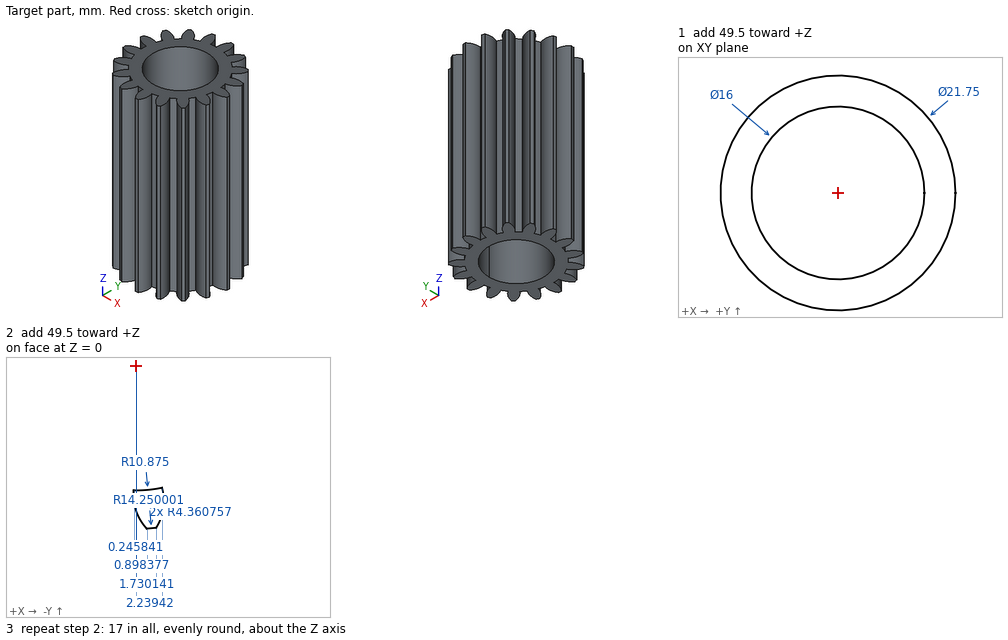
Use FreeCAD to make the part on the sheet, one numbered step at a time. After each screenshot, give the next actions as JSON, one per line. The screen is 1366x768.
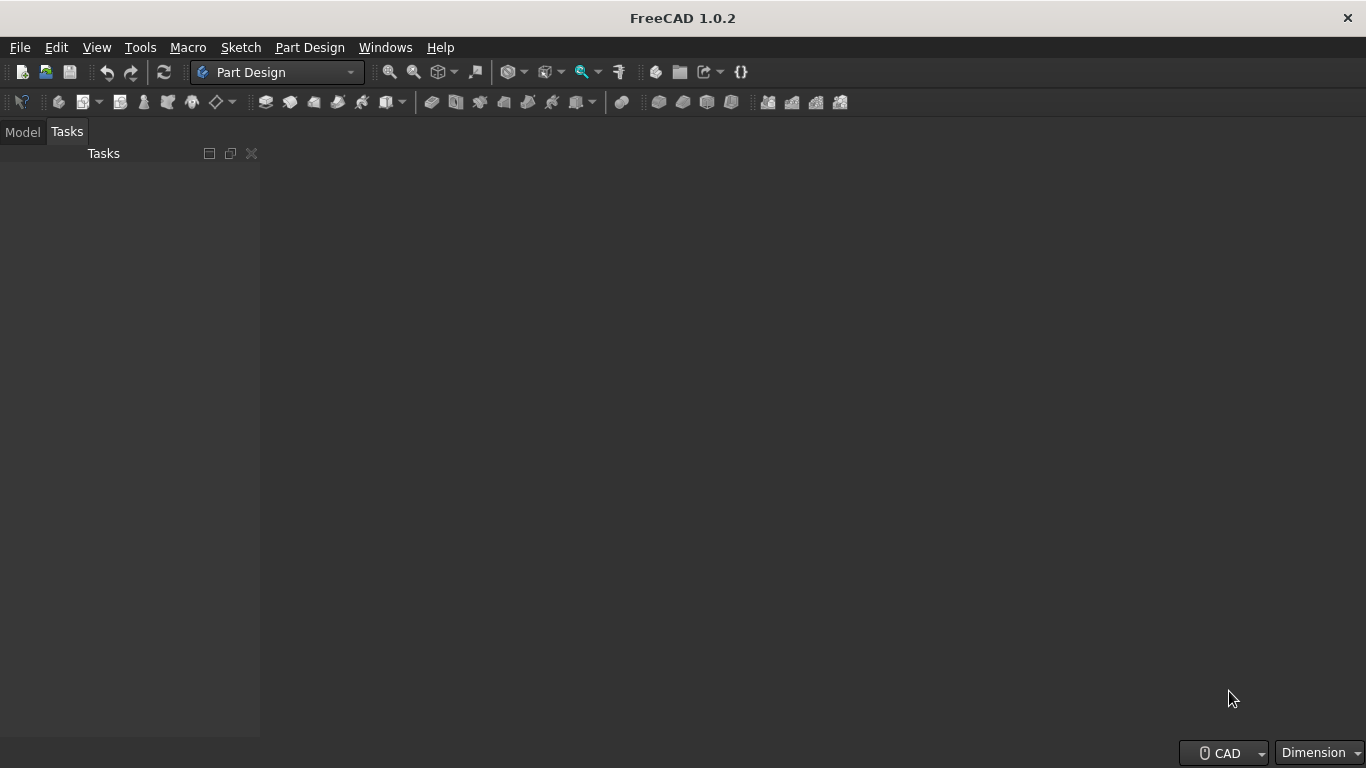
{"action": "left_click", "coordinate": [22, 72]}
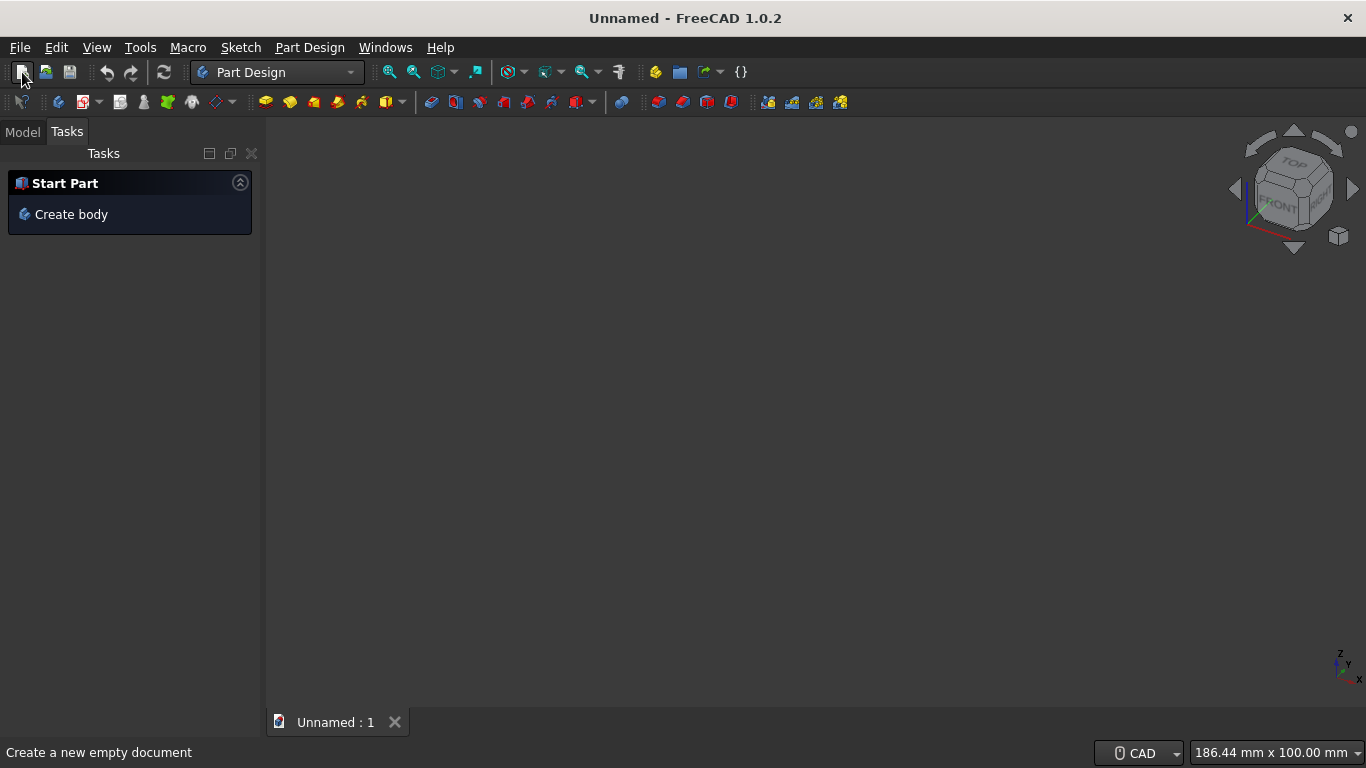
{"action": "left_click", "coordinate": [84, 102]}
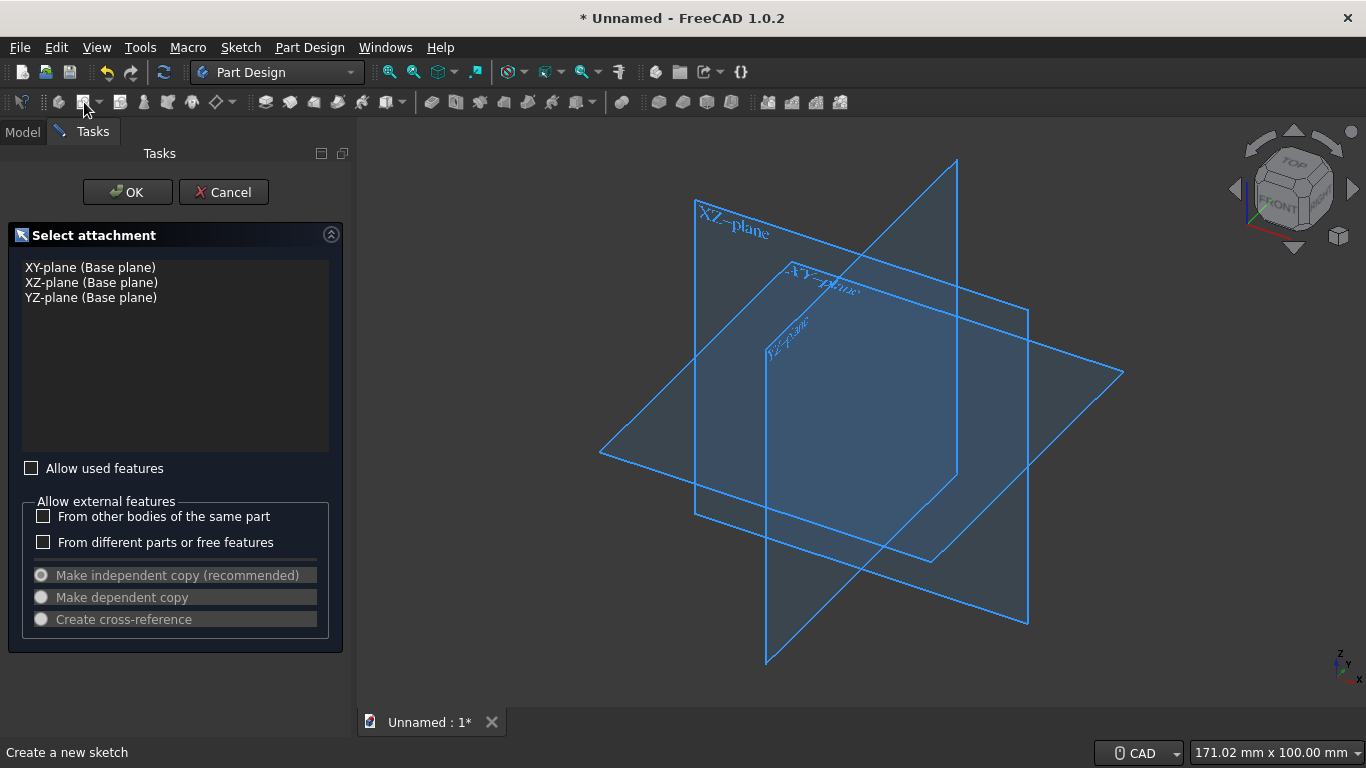
{"action": "left_click", "coordinate": [82, 268]}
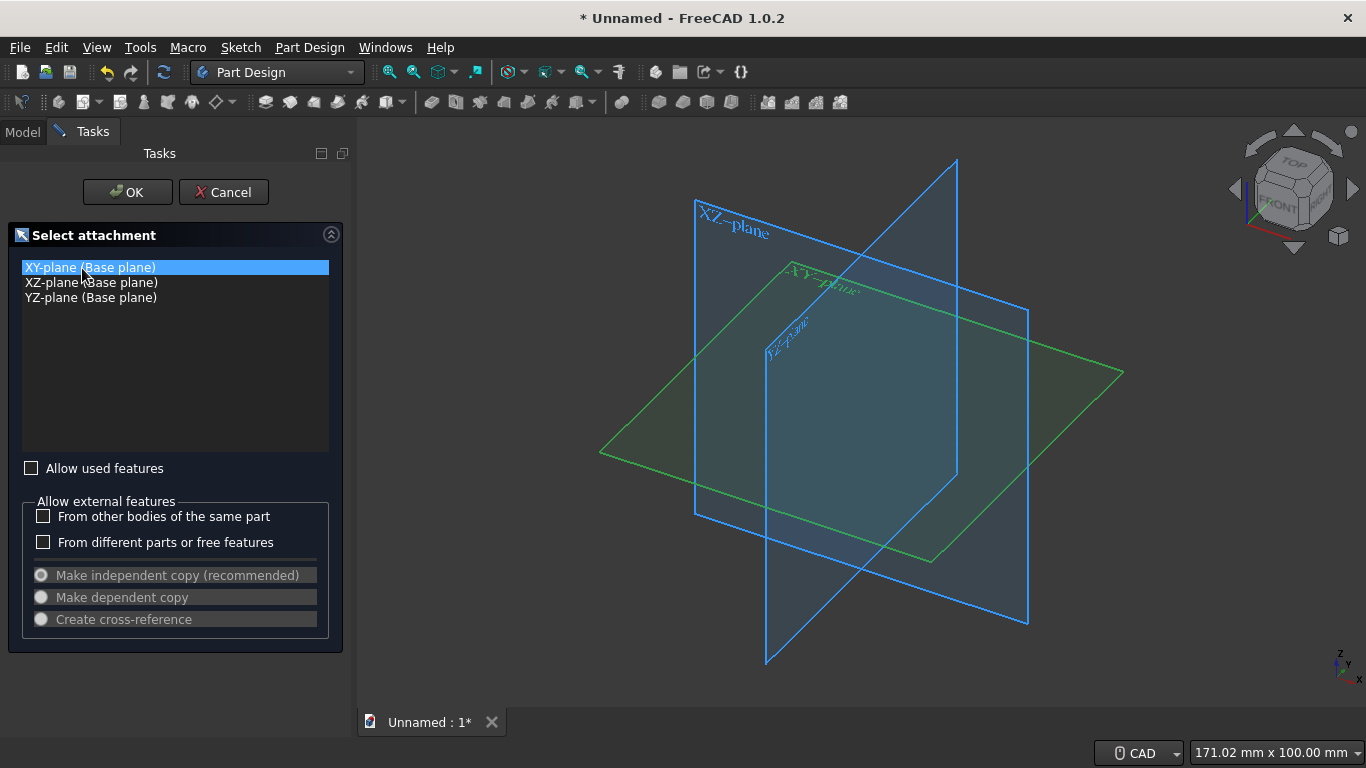
{"action": "left_click", "coordinate": [128, 192]}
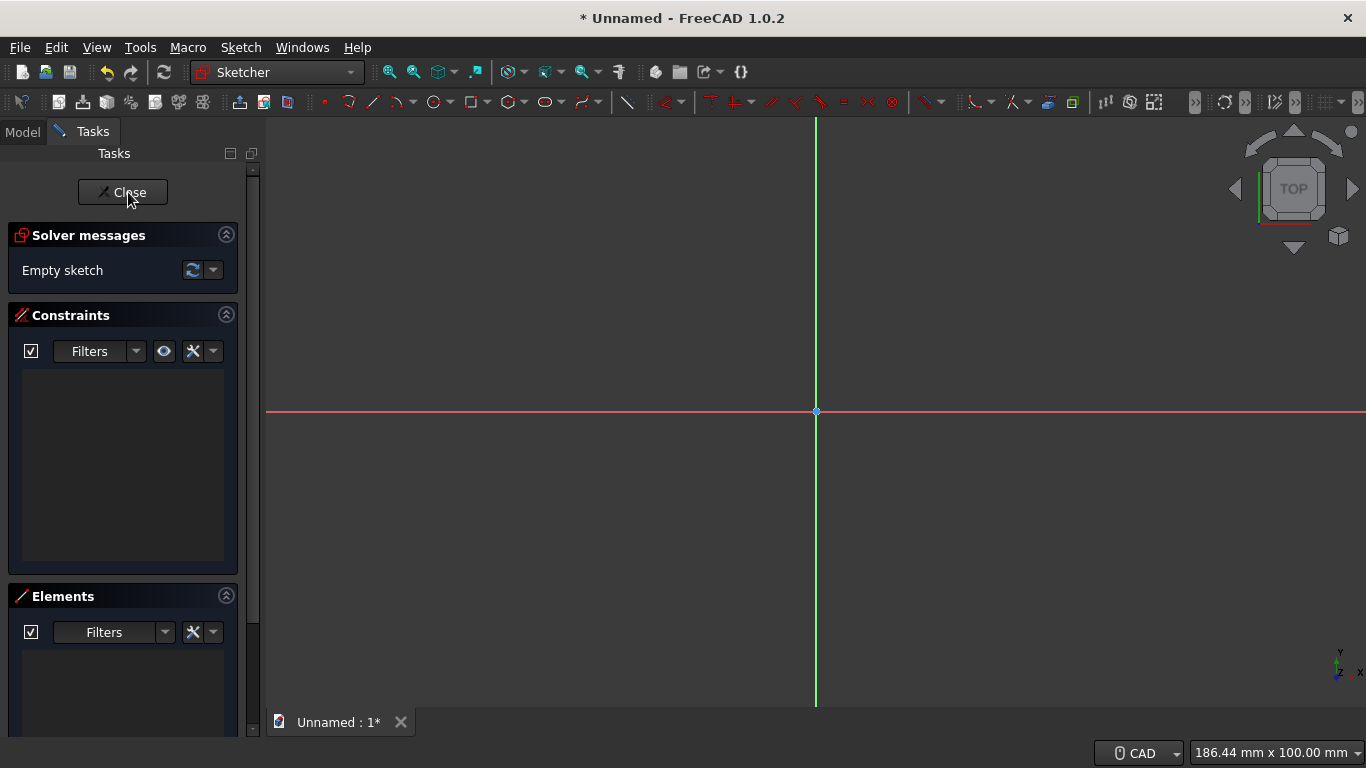
{"action": "scroll", "coordinate": [856, 412], "scroll_direction": "up", "scroll_amount": 5}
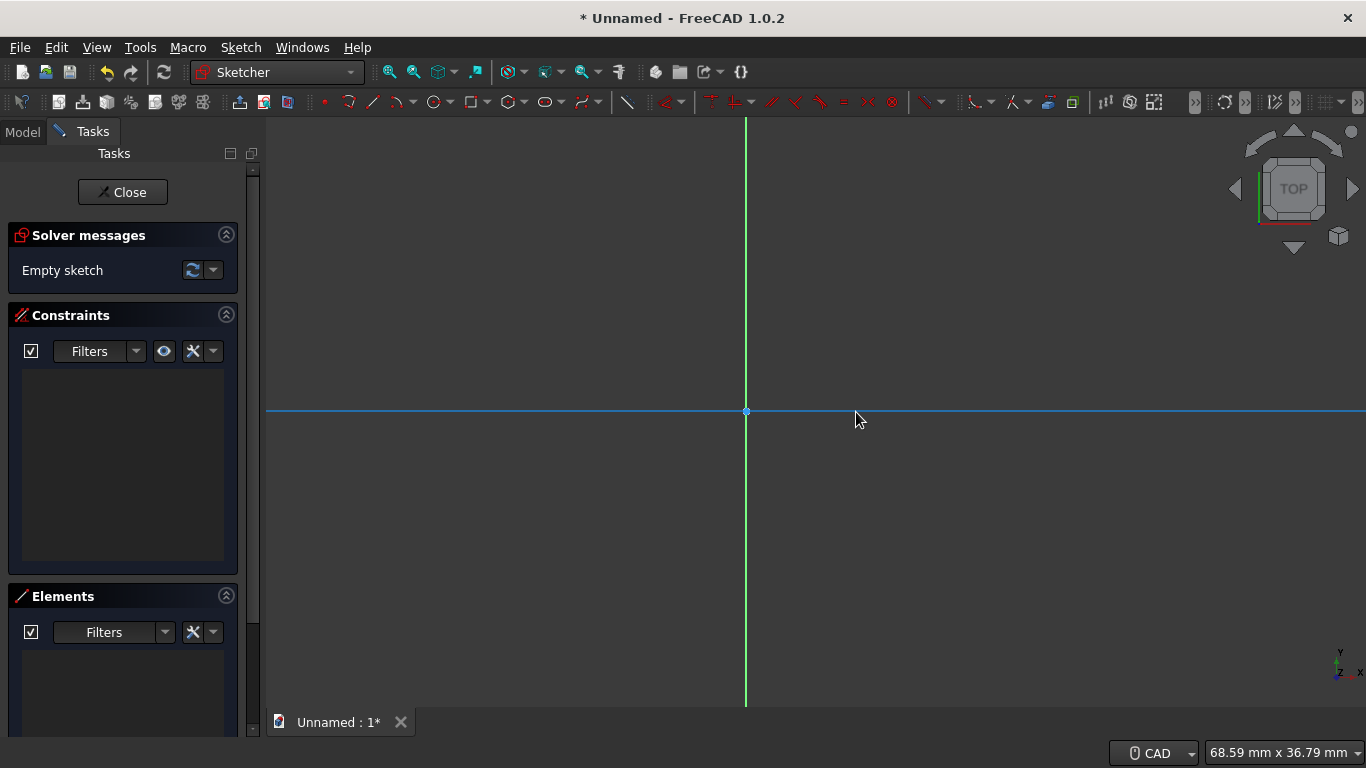
{"action": "left_click", "coordinate": [434, 102]}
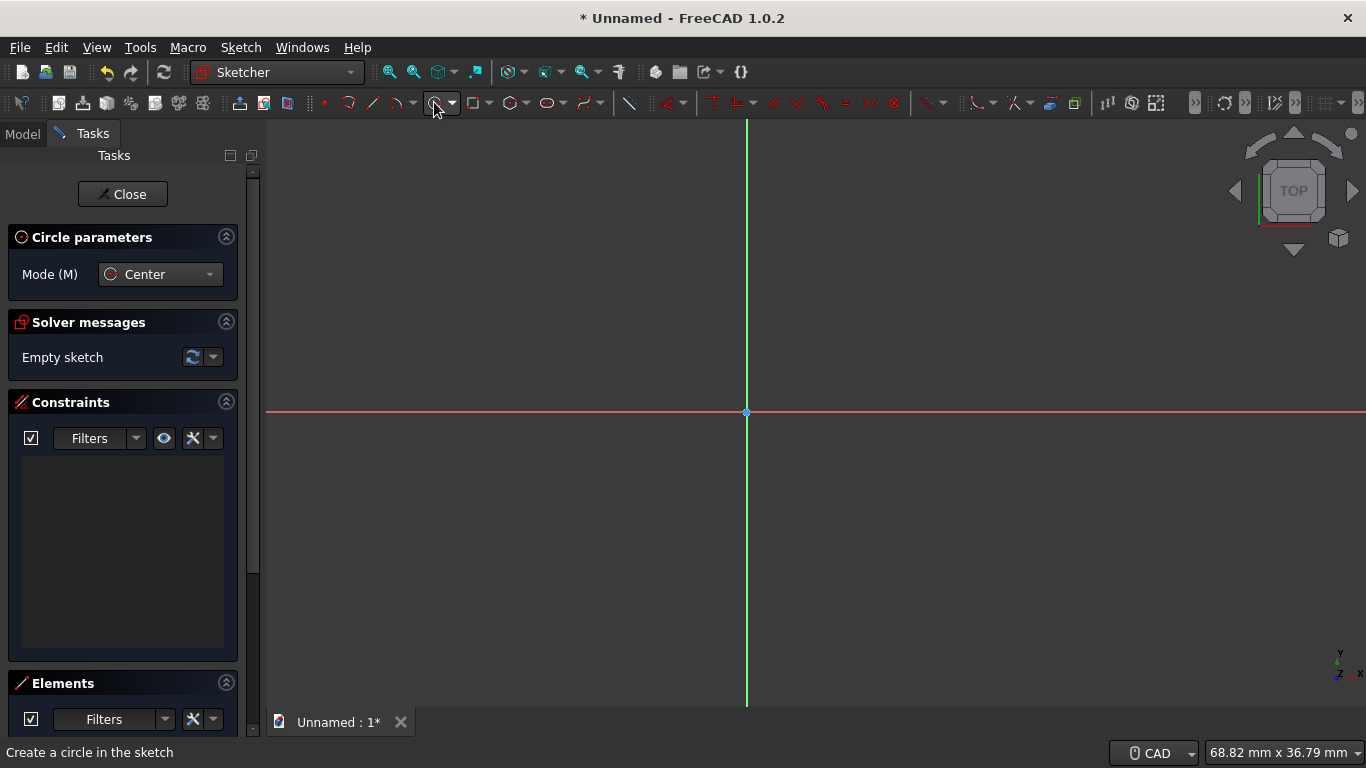
{"action": "left_click", "coordinate": [747, 412]}
{"action": "left_click", "coordinate": [869, 289]}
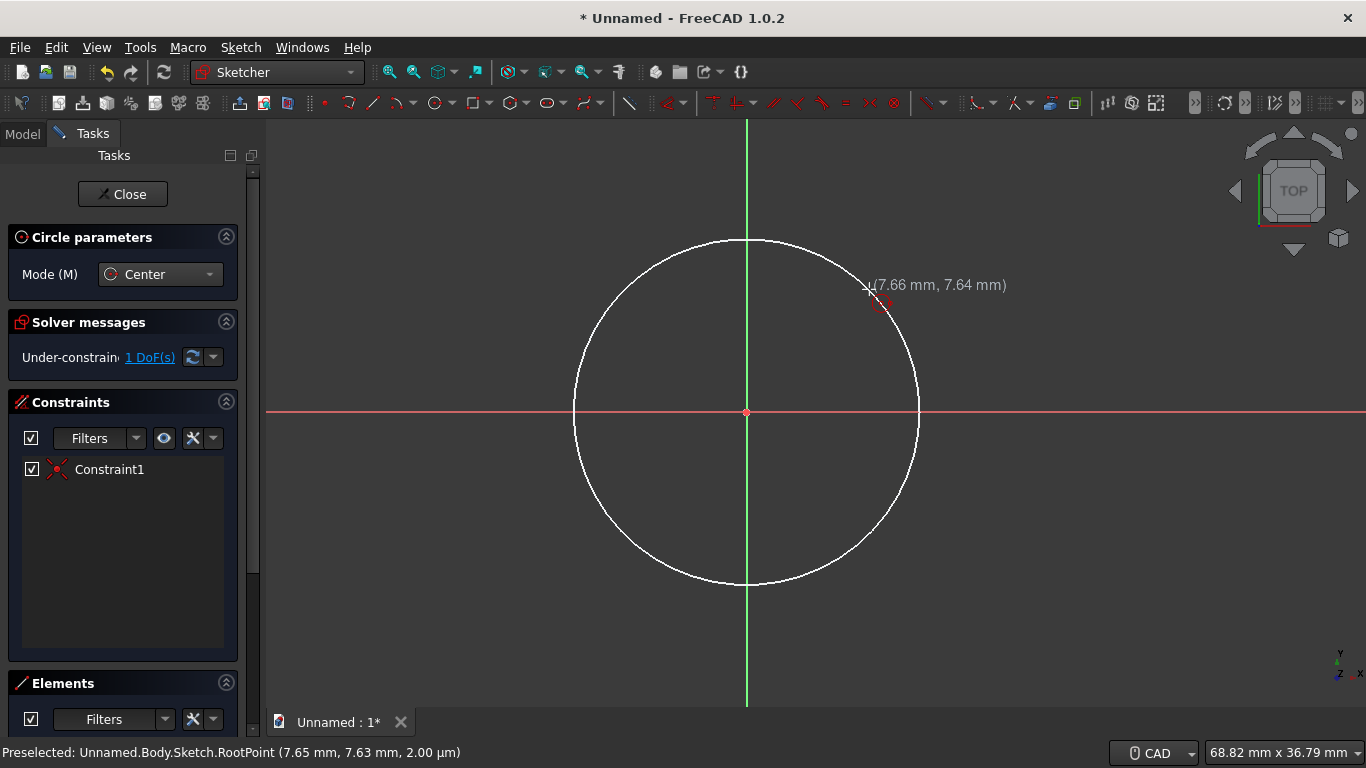
{"action": "left_click", "coordinate": [747, 412]}
{"action": "left_click", "coordinate": [837, 322]}
{"action": "key", "text": "Escape"}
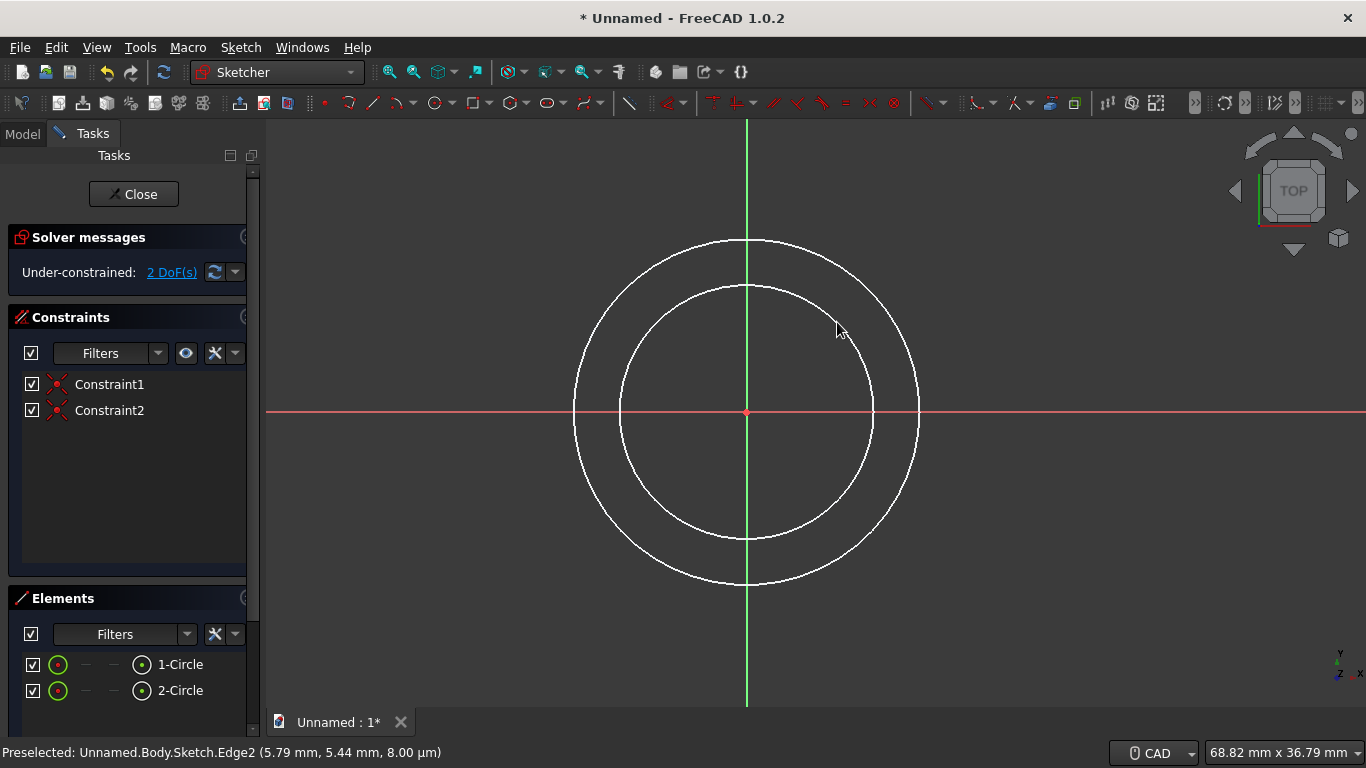
{"action": "left_click", "coordinate": [668, 104]}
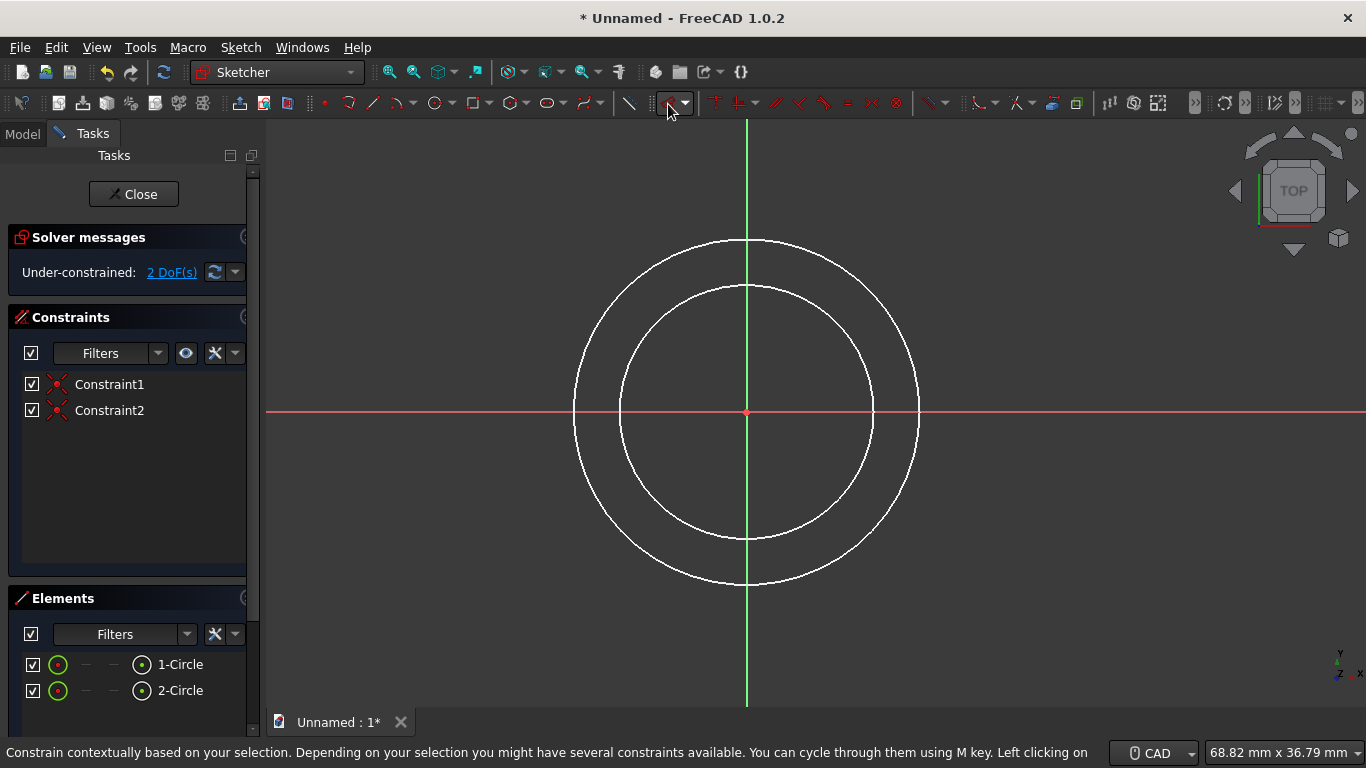
{"action": "left_click", "coordinate": [868, 289]}
{"action": "left_click", "coordinate": [890, 266]}